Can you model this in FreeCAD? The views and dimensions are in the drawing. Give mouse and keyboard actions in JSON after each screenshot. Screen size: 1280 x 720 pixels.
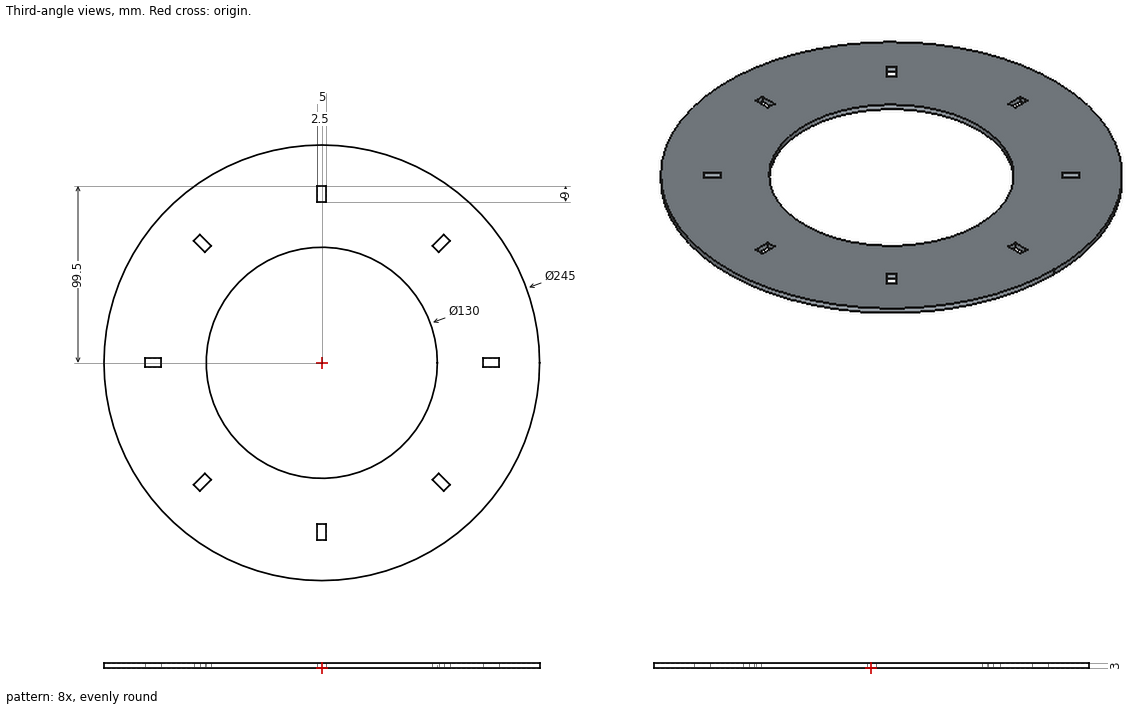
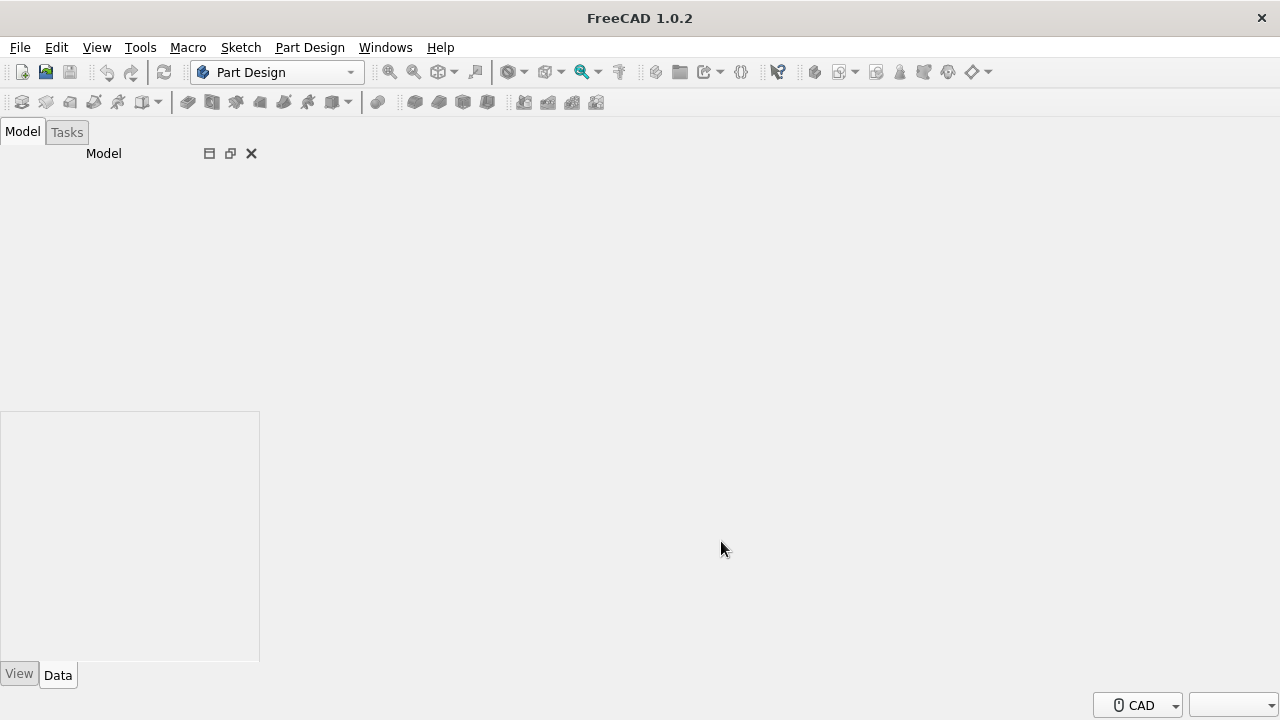
{"action": "key", "text": "ctrl+n"}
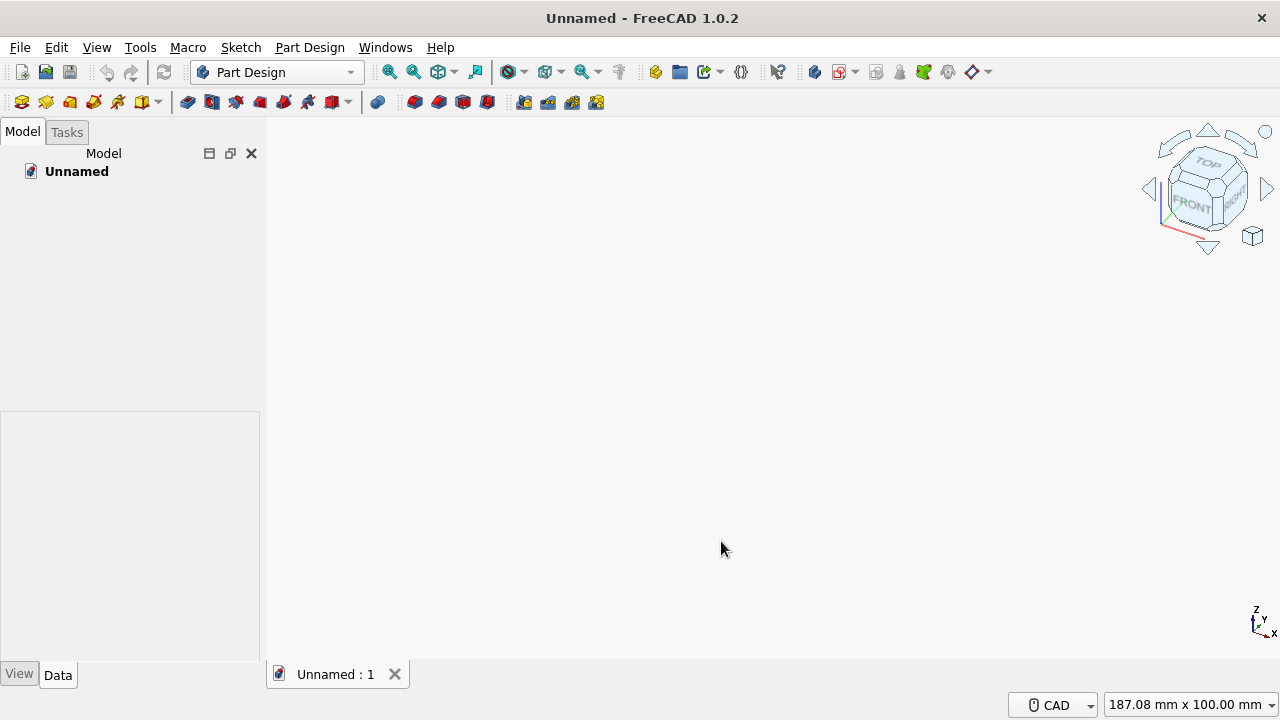
{"action": "left_click", "coordinate": [840, 72]}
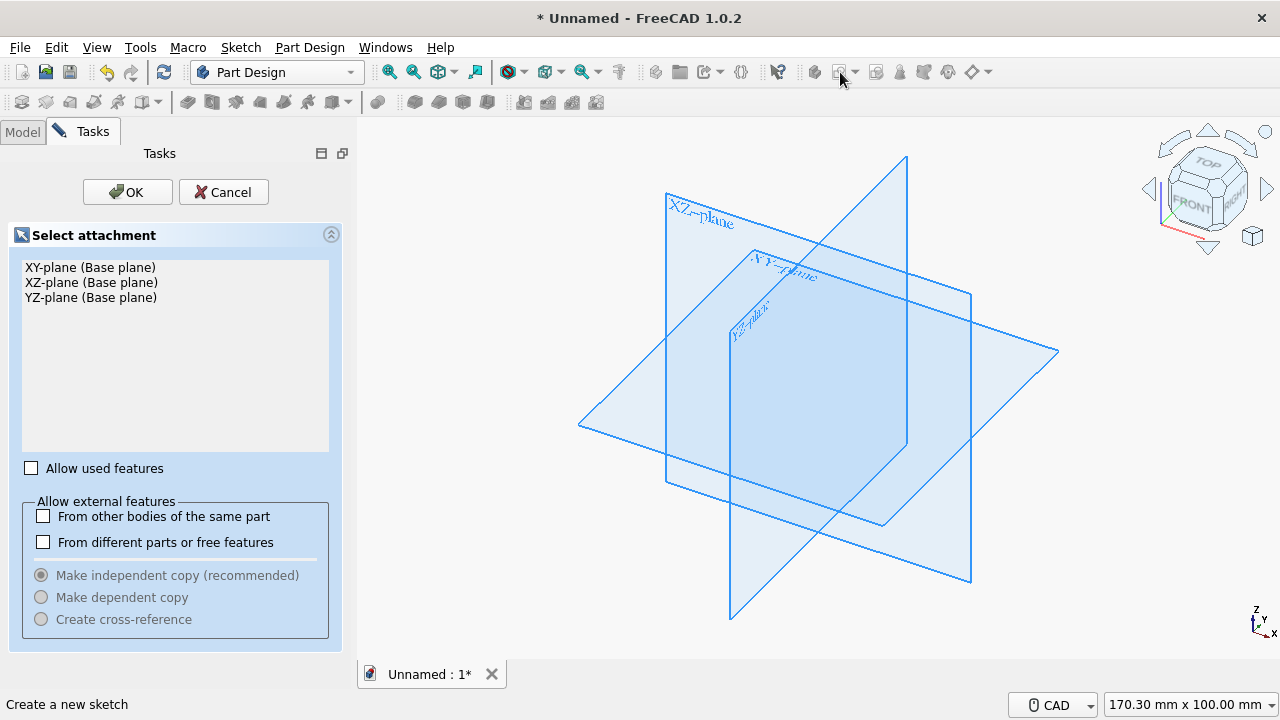
{"action": "left_click", "coordinate": [82, 268]}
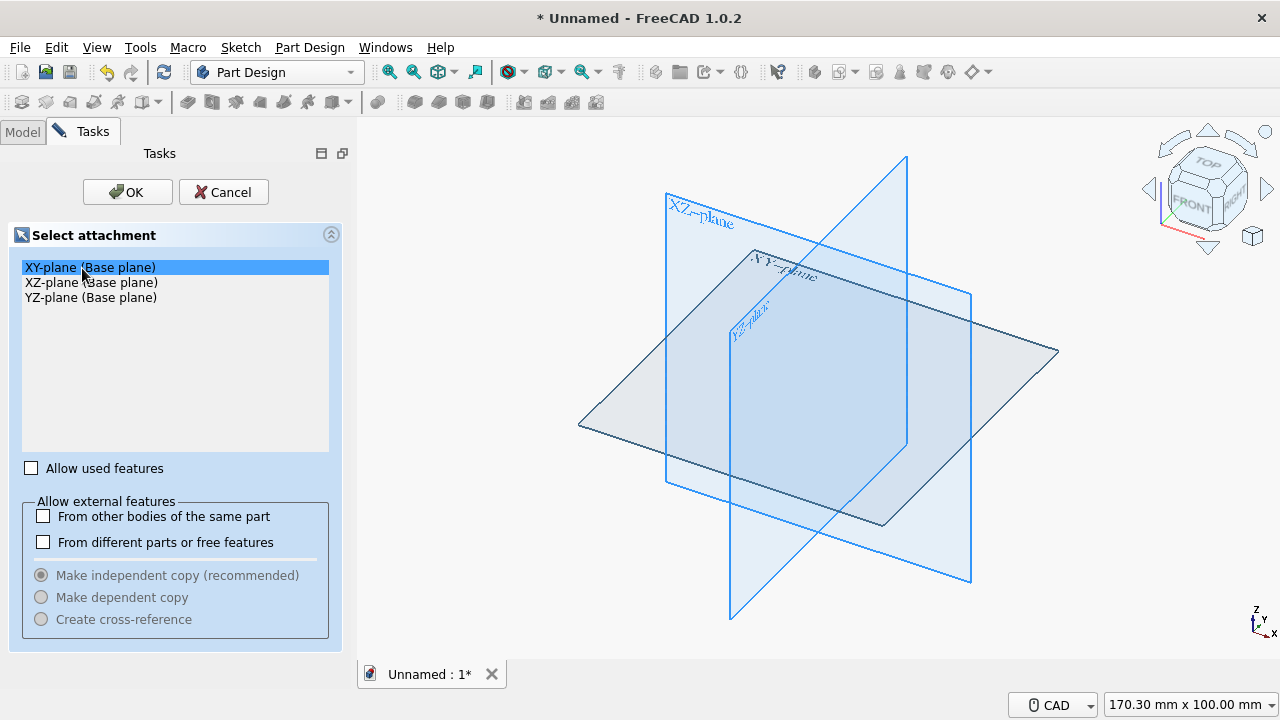
{"action": "left_click", "coordinate": [128, 192]}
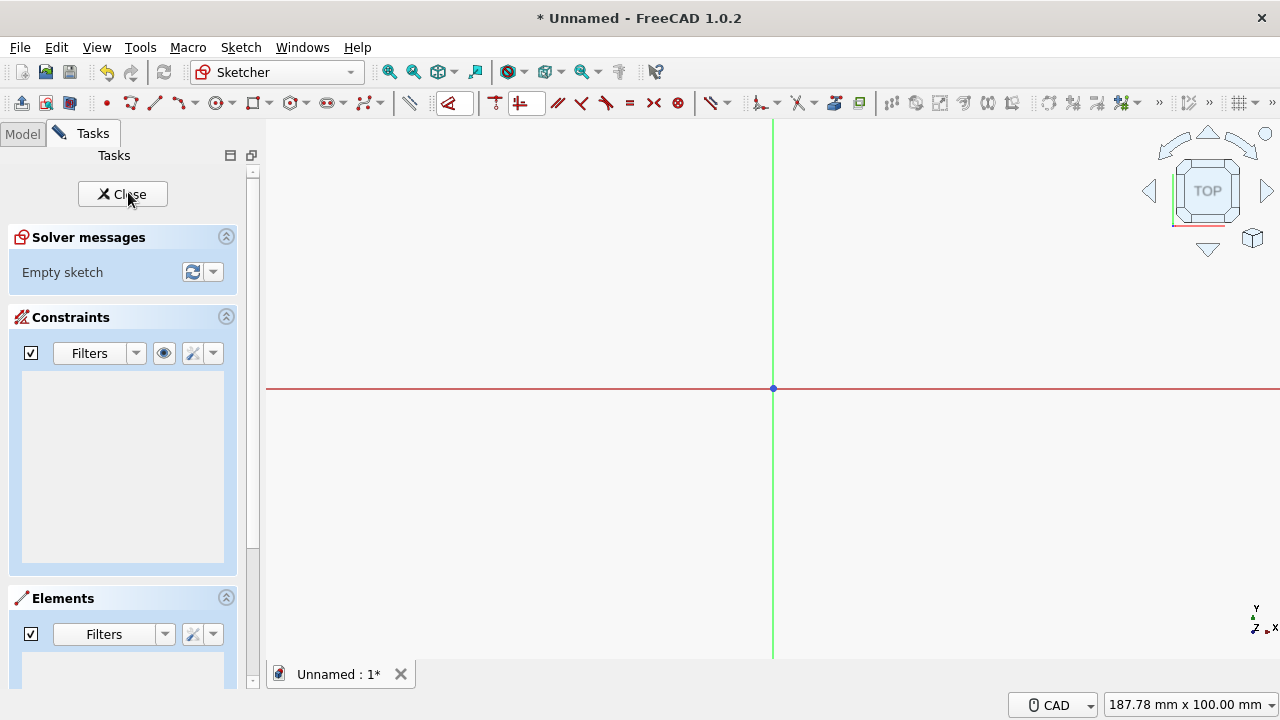
{"action": "scroll", "coordinate": [682, 389], "scroll_direction": "down", "scroll_amount": 7}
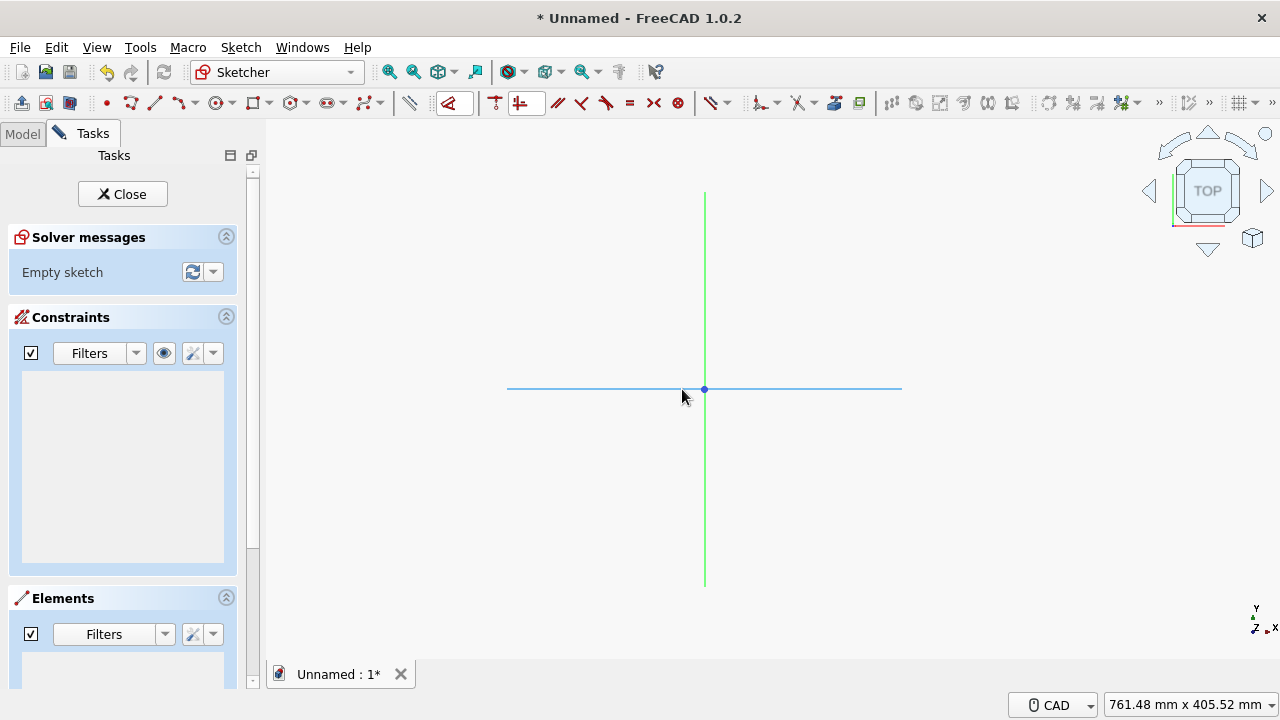
{"action": "key", "text": "g c"}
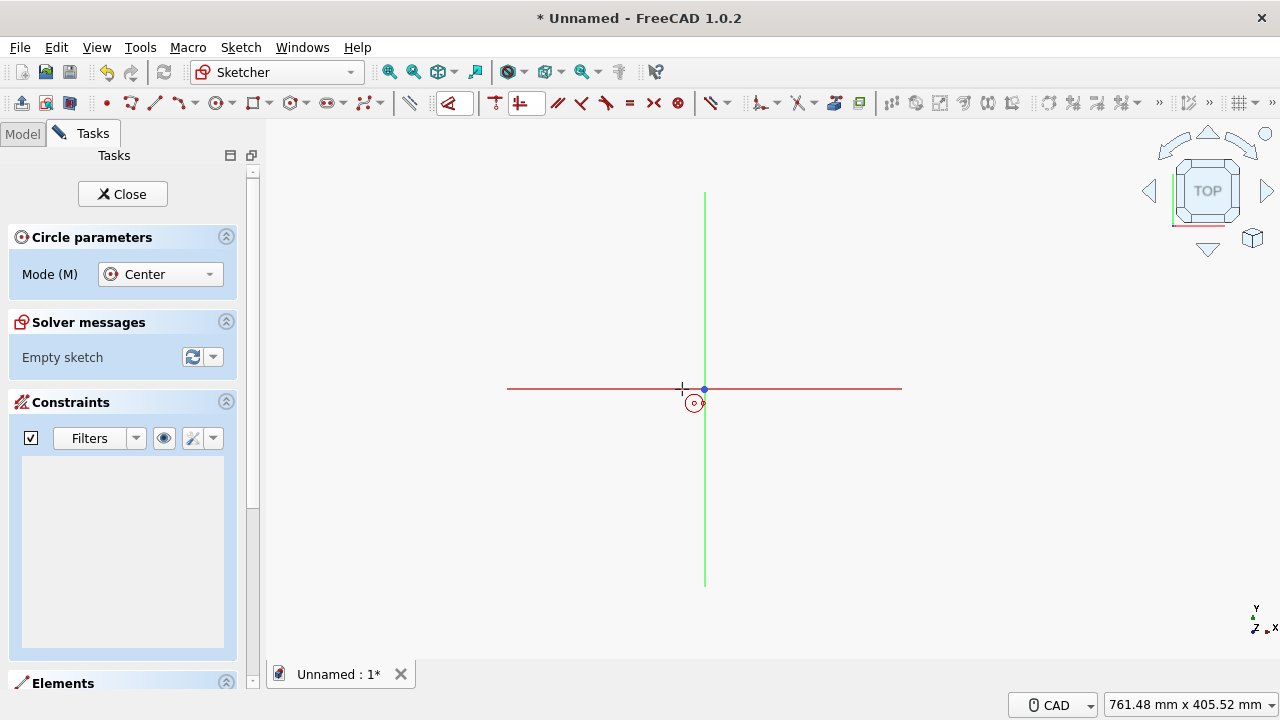
{"action": "left_click", "coordinate": [705, 389]}
{"action": "mouse_move", "coordinate": [820, 274]}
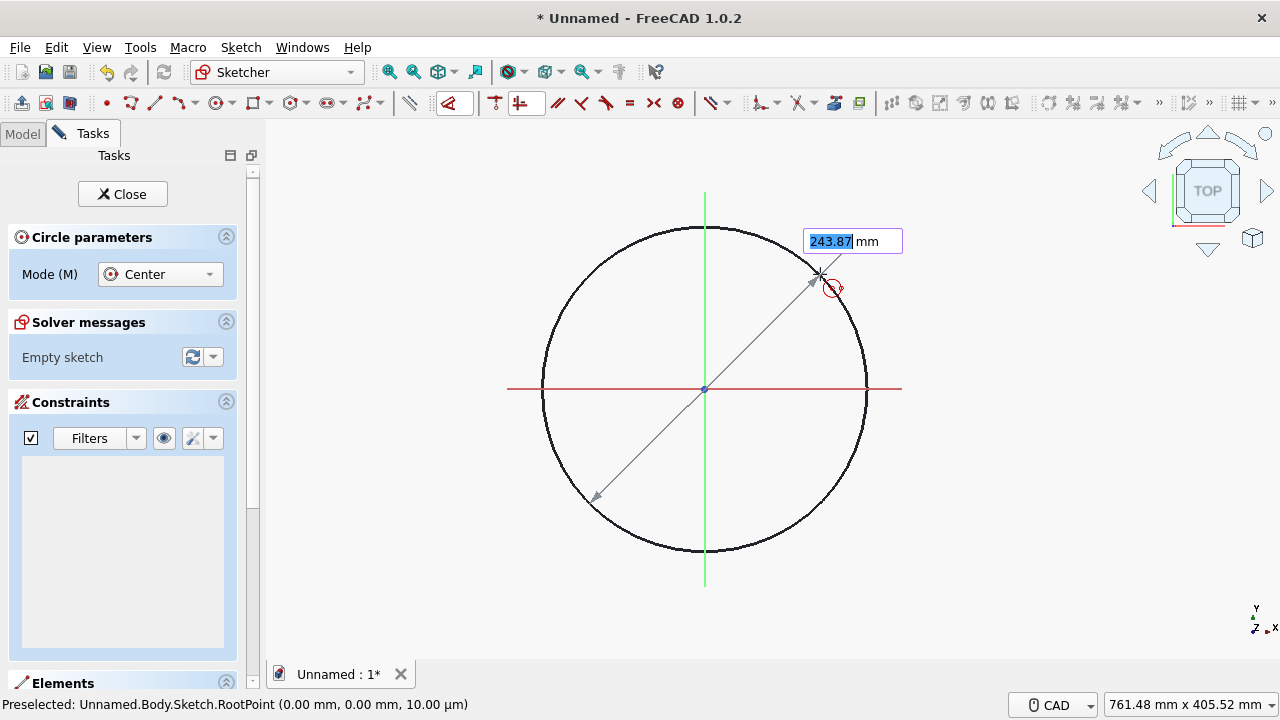
{"action": "type", "text": "245"}
{"action": "key", "text": "Return"}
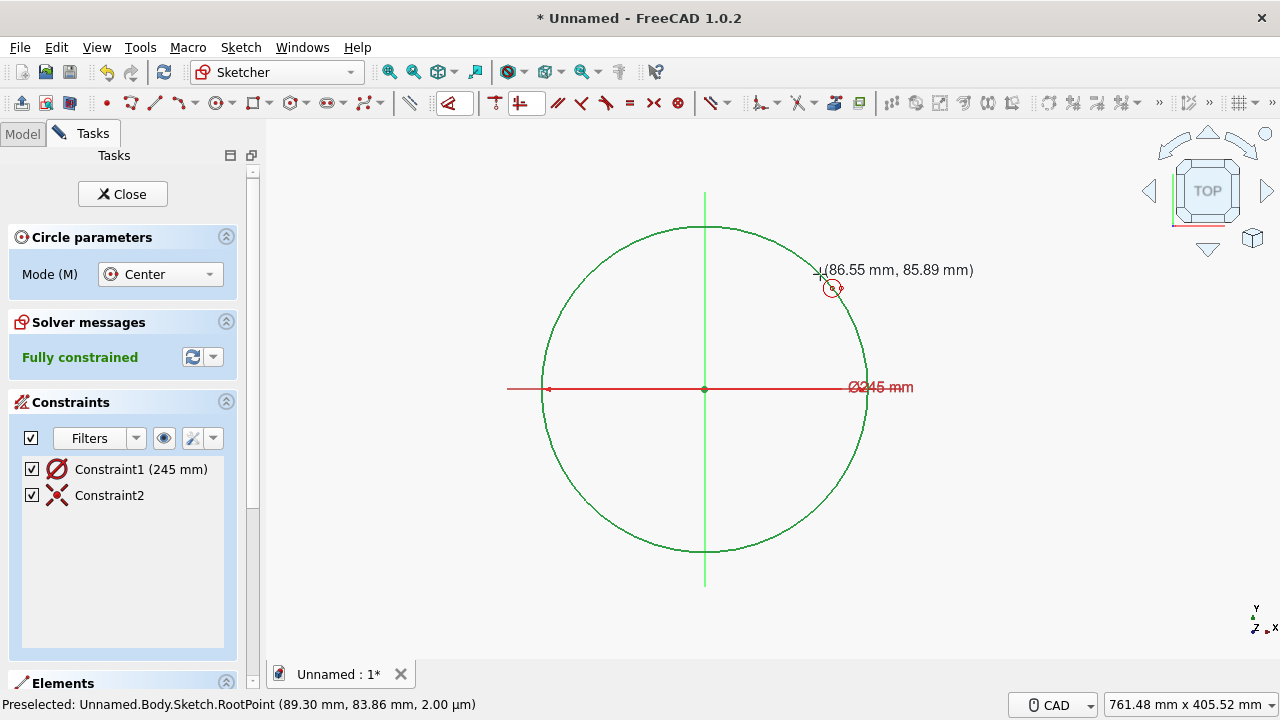
{"action": "left_click", "coordinate": [705, 389]}
{"action": "mouse_move", "coordinate": [766, 328]}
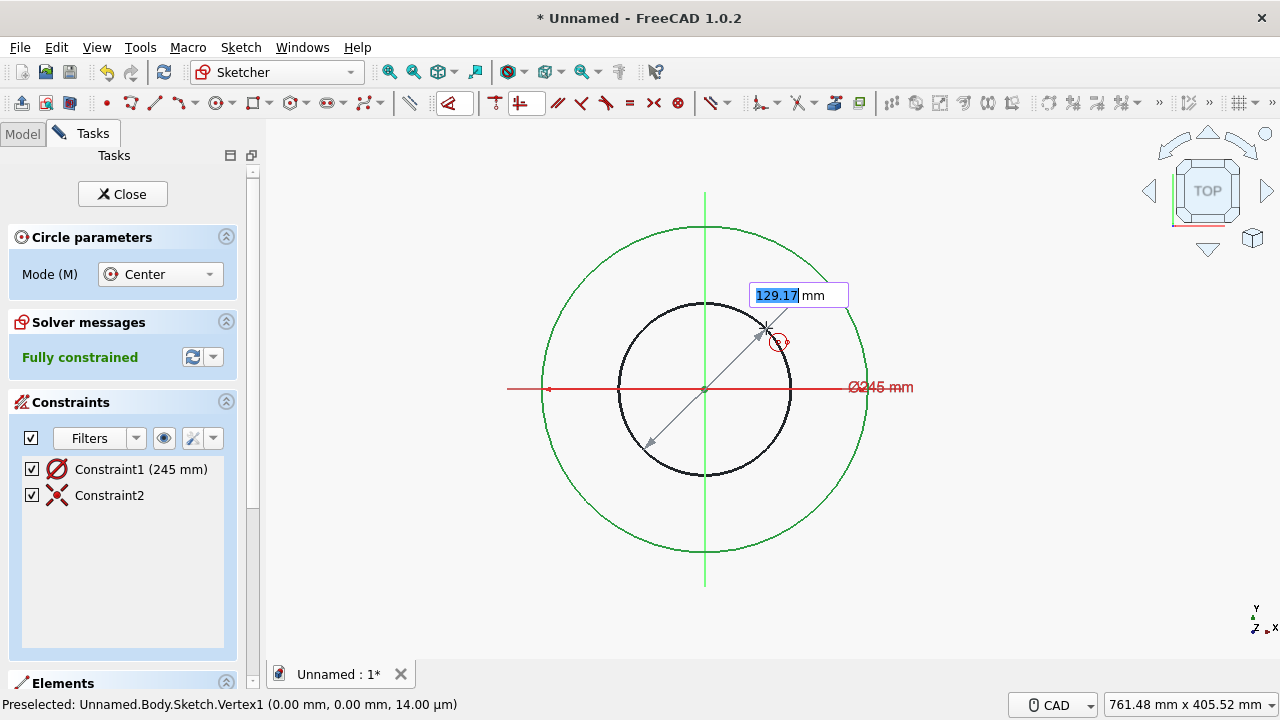
{"action": "type", "text": "130"}
{"action": "key", "text": "Return"}
{"action": "key", "text": "Escape"}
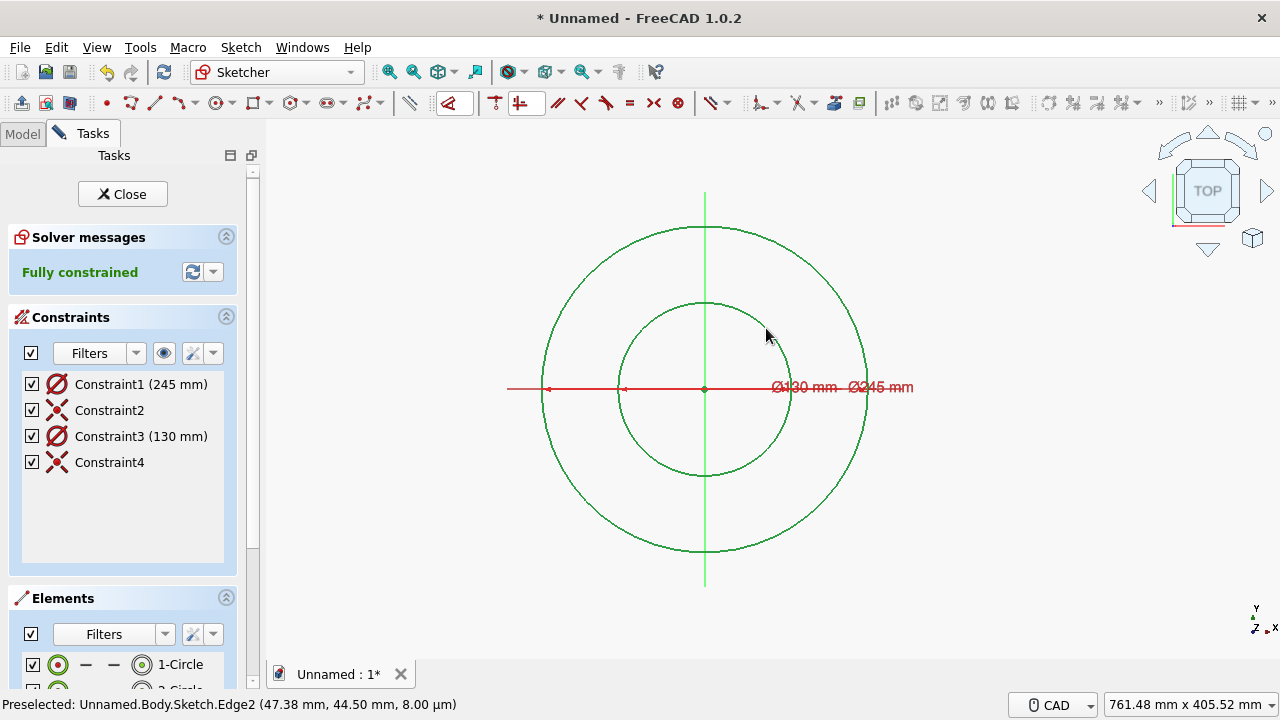
{"action": "left_click", "coordinate": [123, 194]}